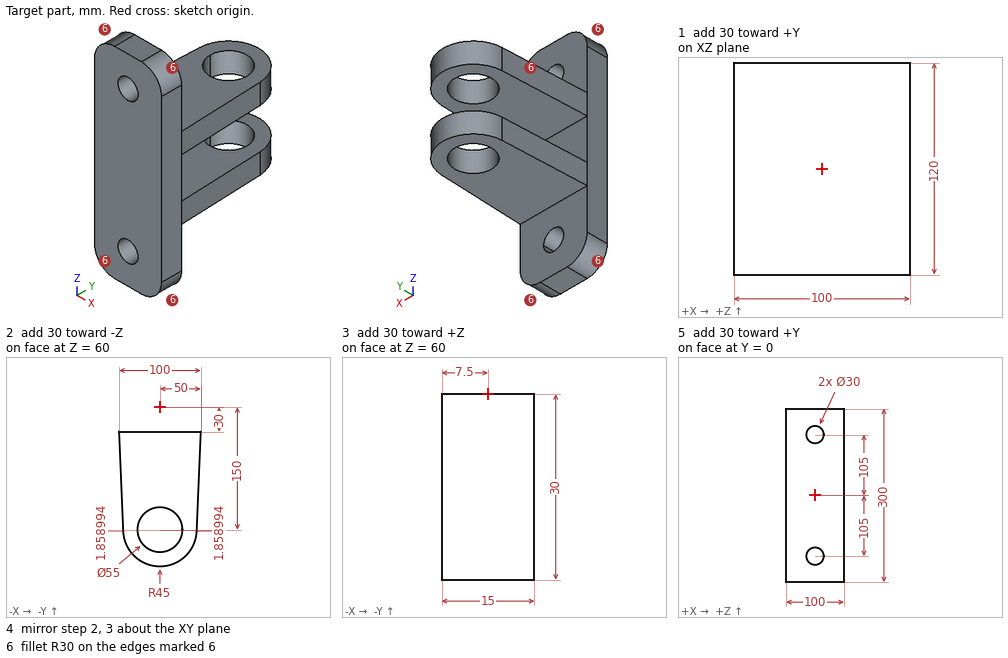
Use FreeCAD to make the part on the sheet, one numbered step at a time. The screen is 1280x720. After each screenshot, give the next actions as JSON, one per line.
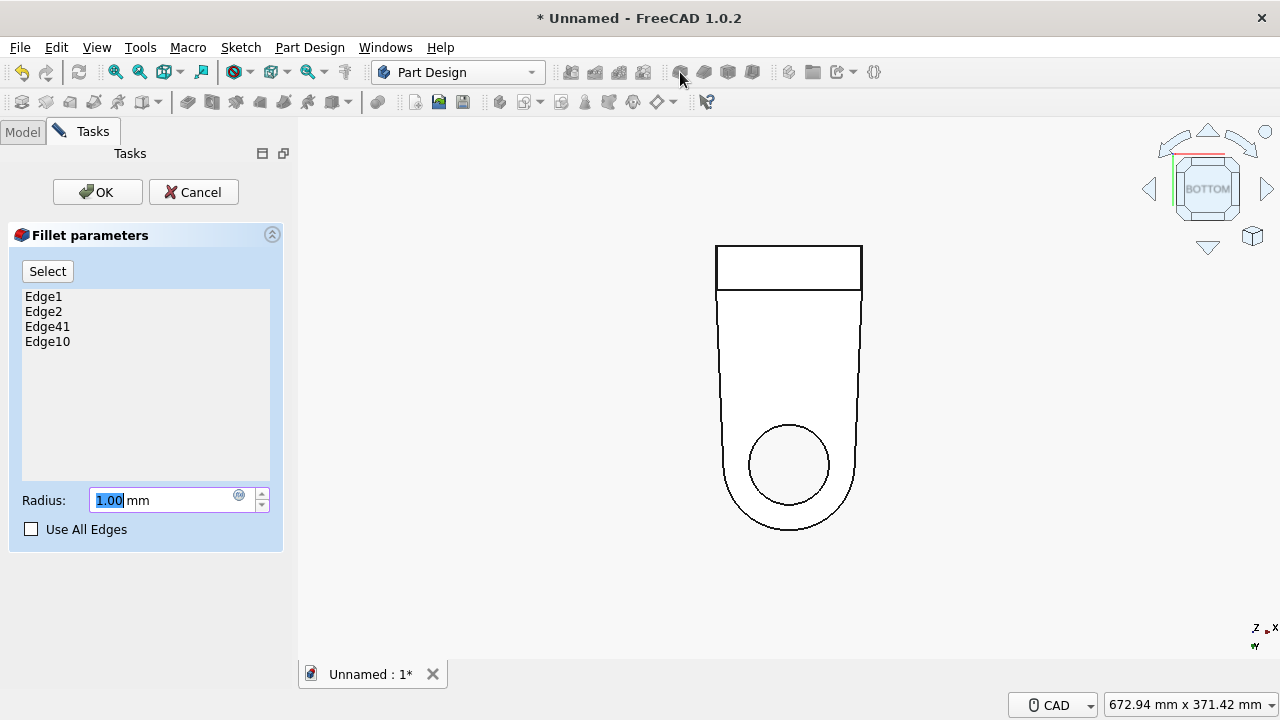
{"action": "type", "text": "30"}
{"action": "key", "text": "Tab"}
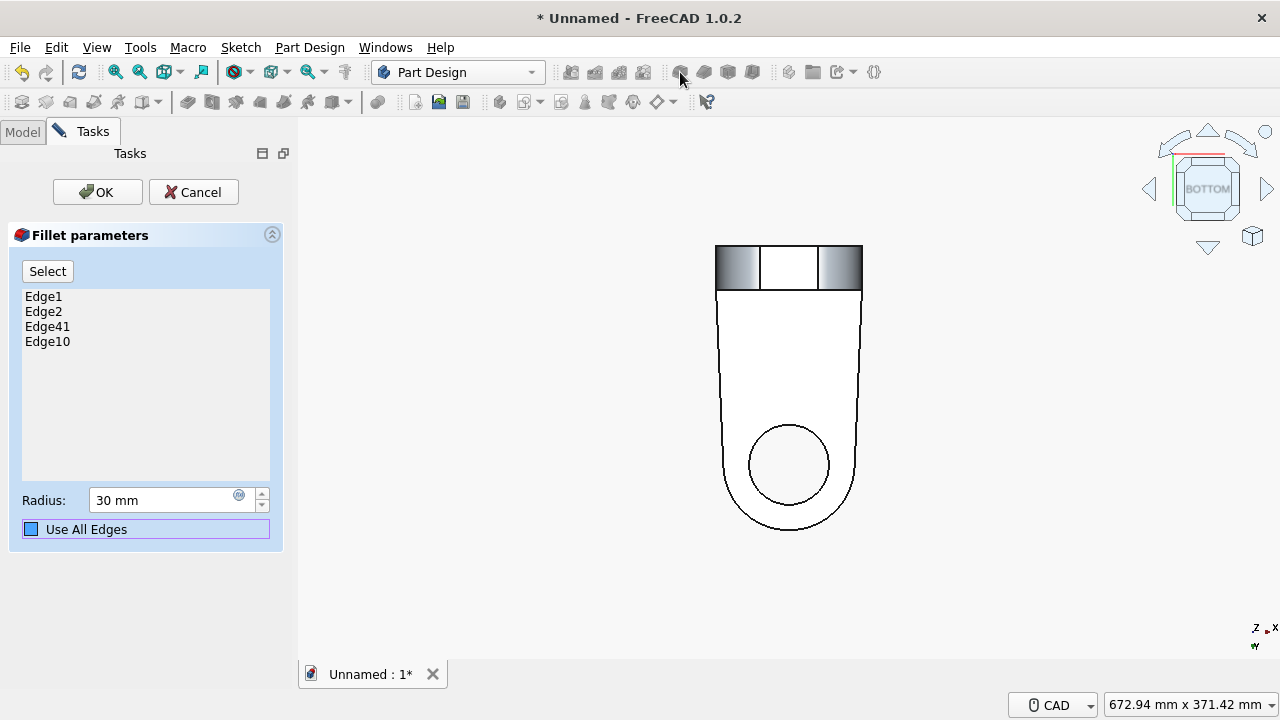
{"action": "left_click", "coordinate": [98, 192]}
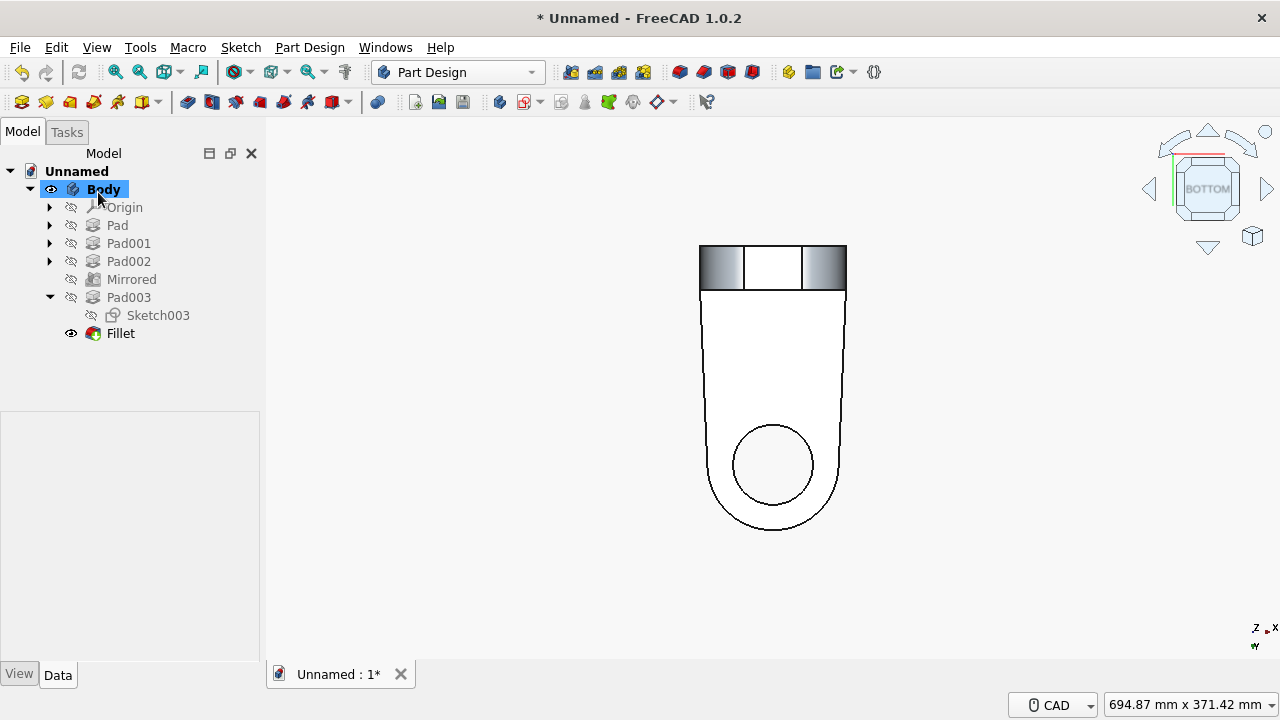
{"action": "key", "text": "0"}